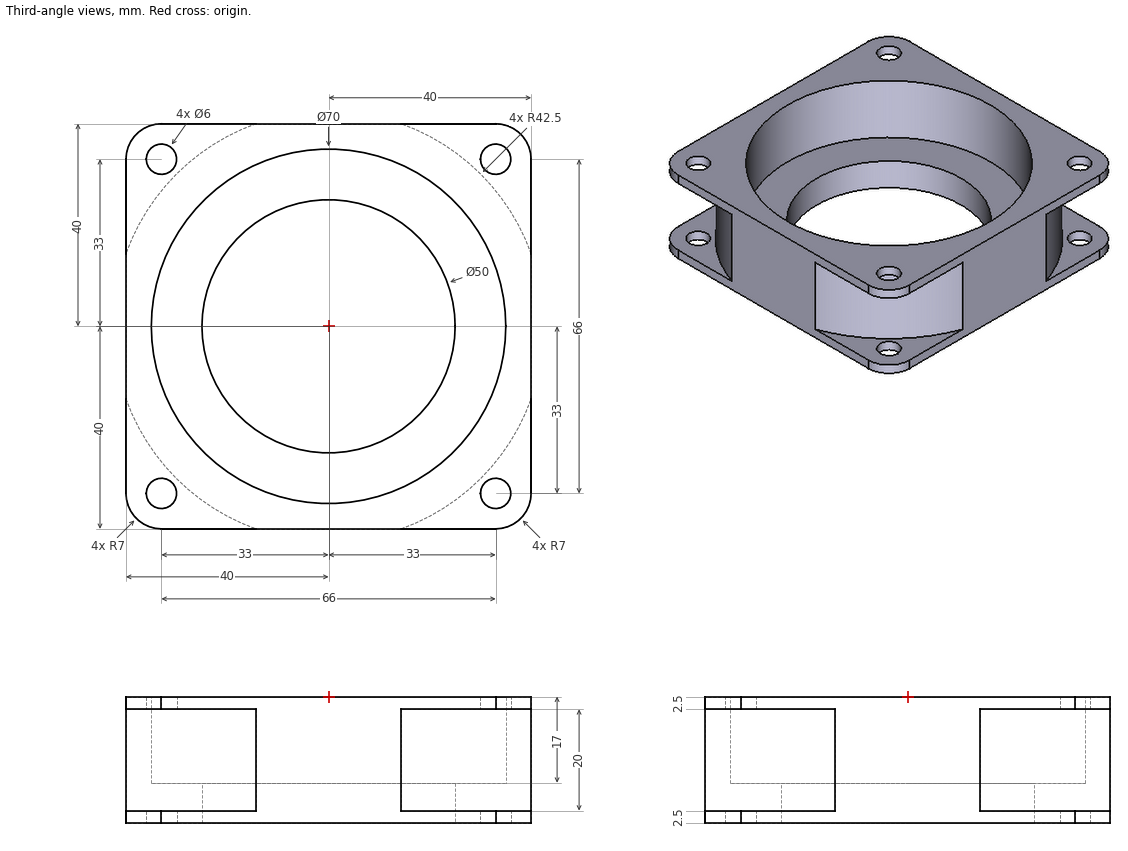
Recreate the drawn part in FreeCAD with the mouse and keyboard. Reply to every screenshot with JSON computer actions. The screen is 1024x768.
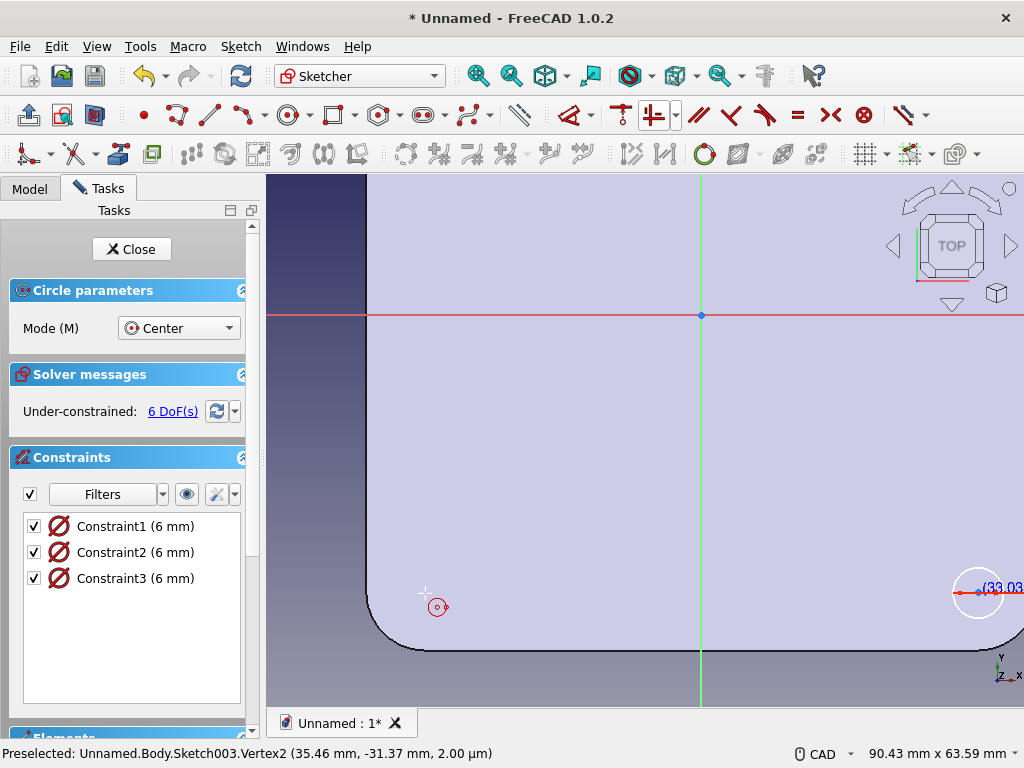
{"action": "left_click", "coordinate": [425, 592]}
{"action": "mouse_move", "coordinate": [443, 574]}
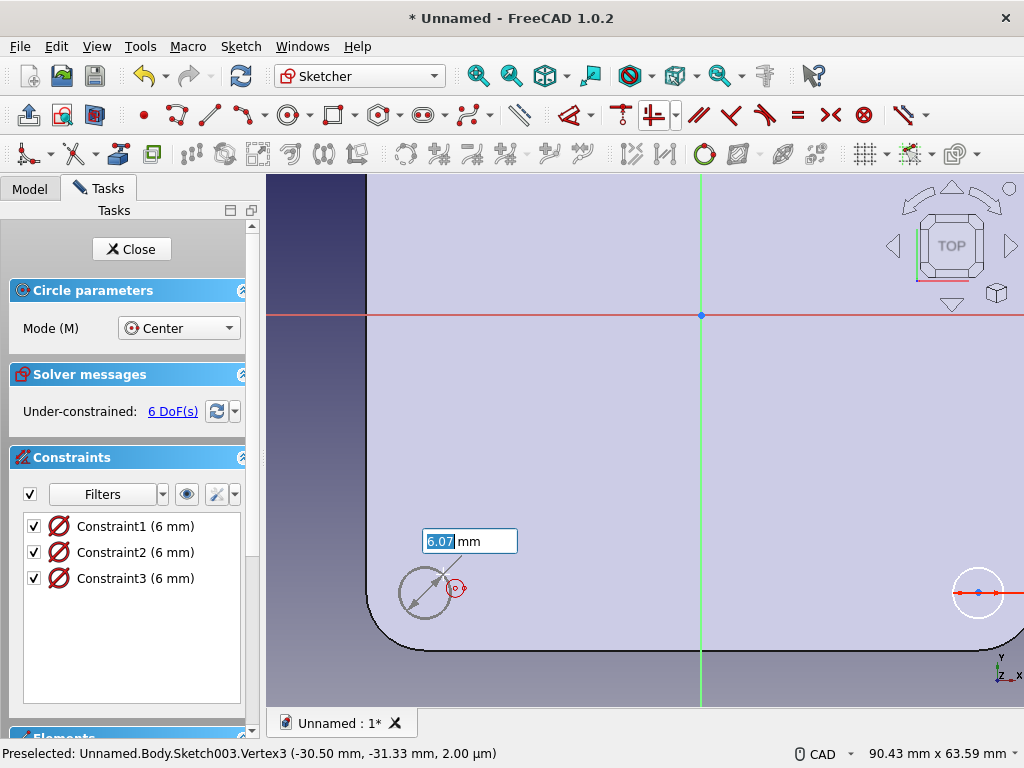
{"action": "type", "text": "6"}
{"action": "key", "text": "Return"}
{"action": "key", "text": "Escape"}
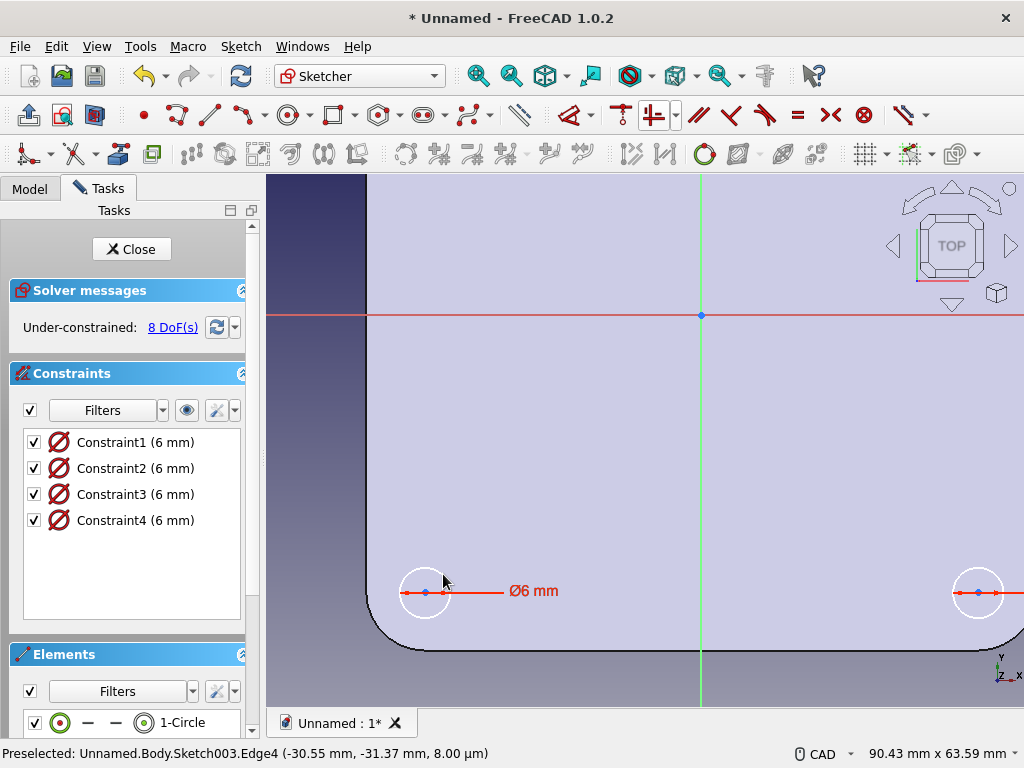
{"action": "scroll", "coordinate": [425, 593], "scroll_direction": "down", "scroll_amount": 3}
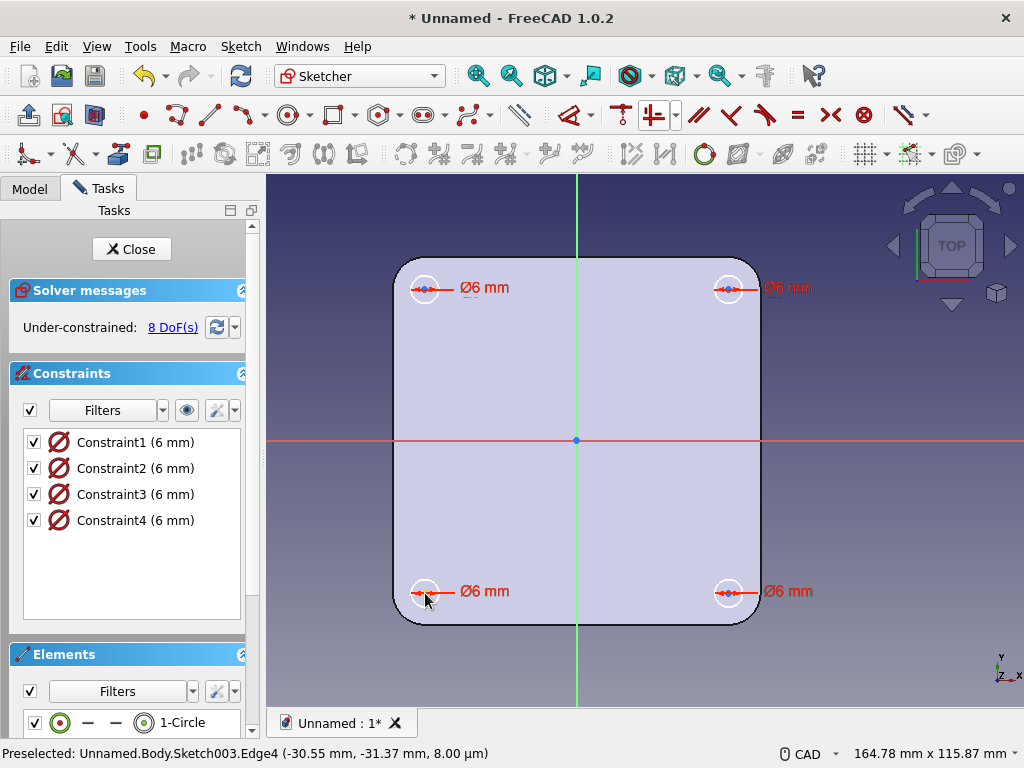
{"action": "left_click", "coordinate": [425, 290]}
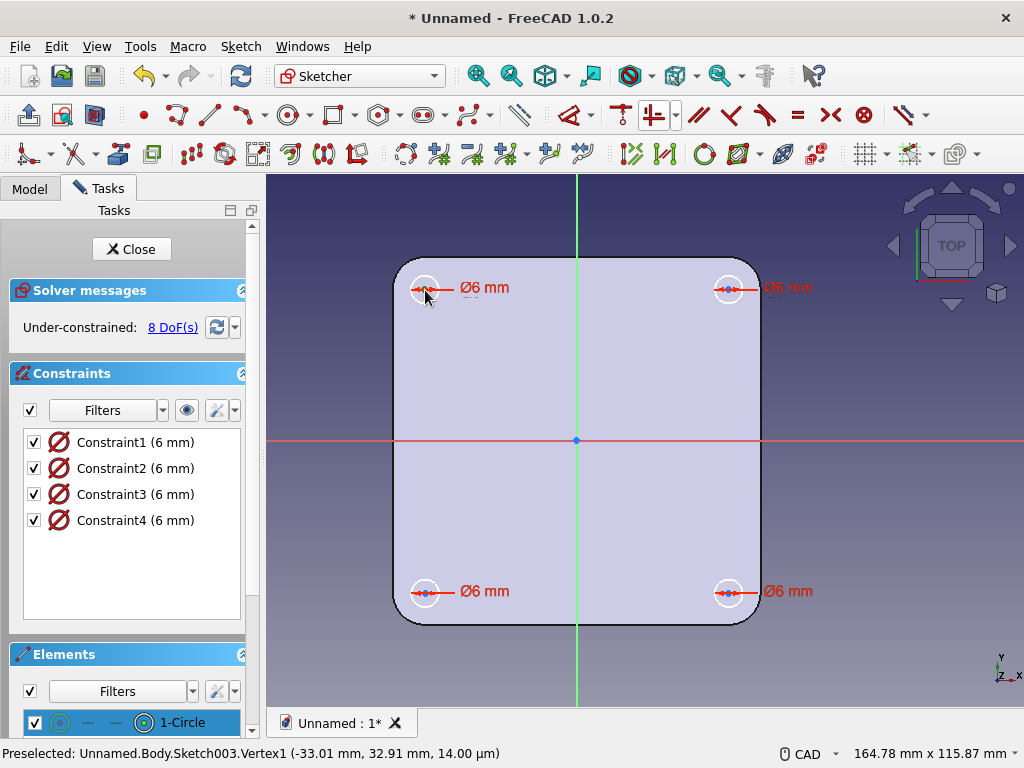
{"action": "left_click", "coordinate": [729, 290]}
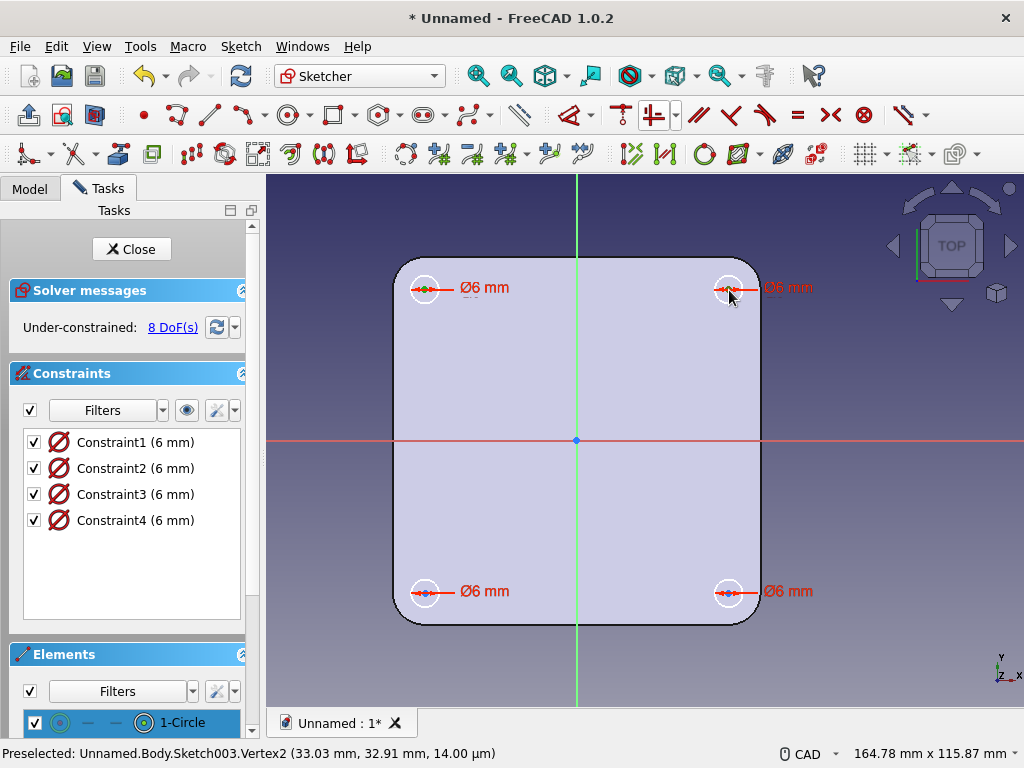
{"action": "key", "text": "h"}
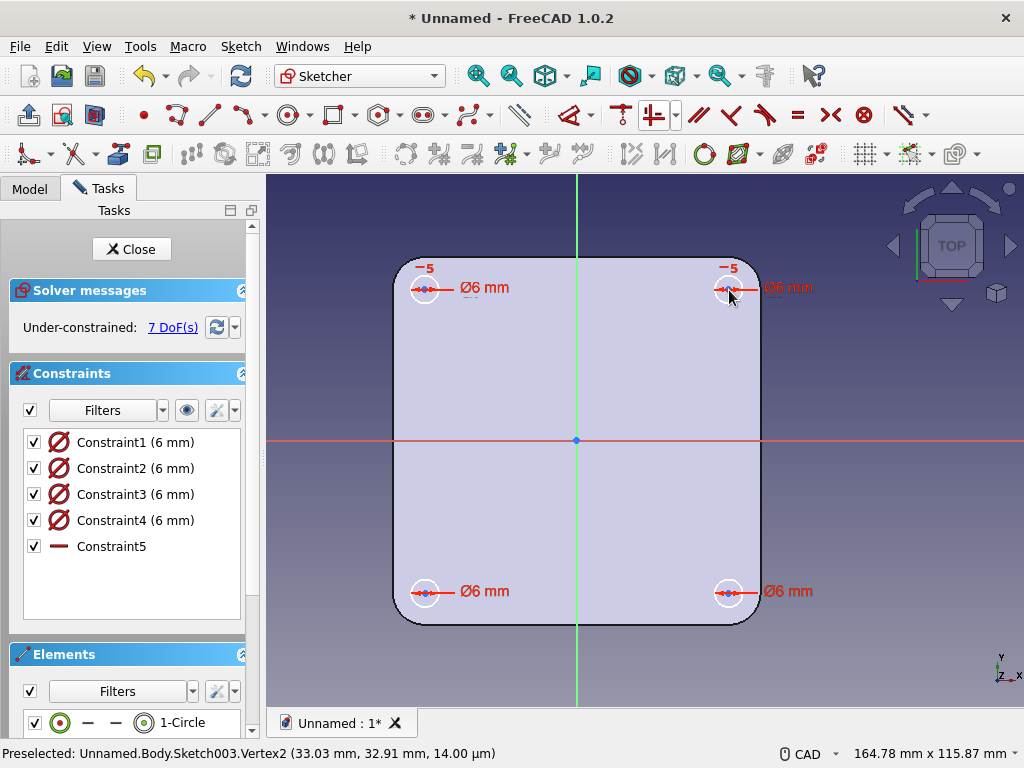
{"action": "left_click", "coordinate": [729, 290]}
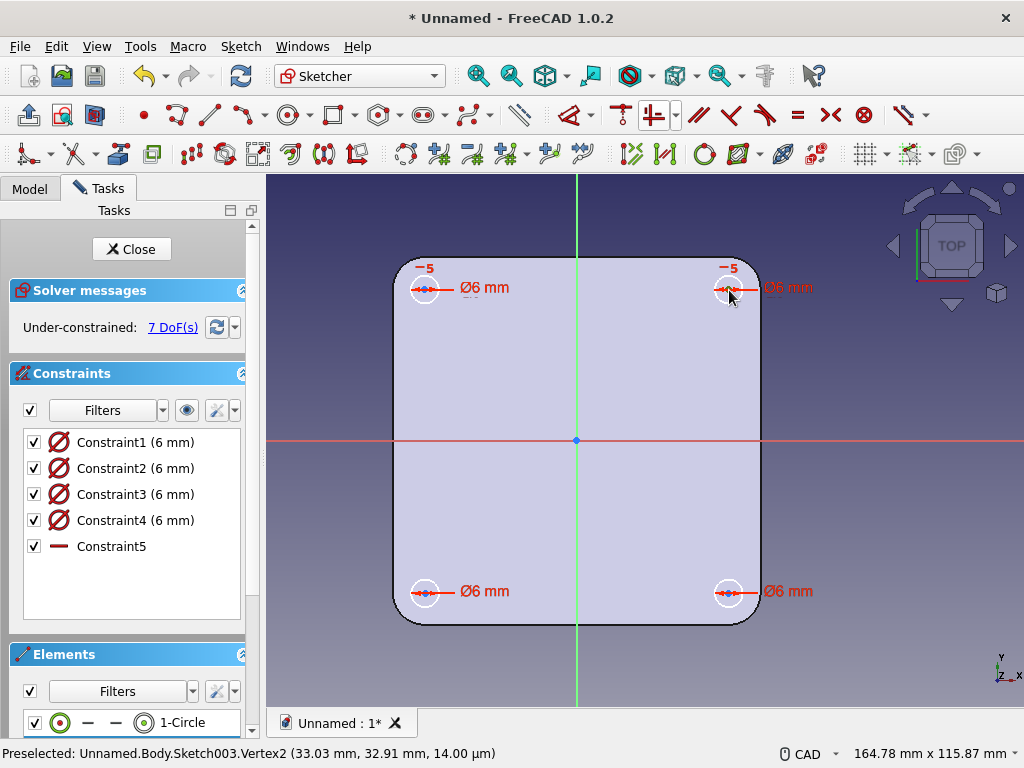
{"action": "left_click", "coordinate": [729, 593]}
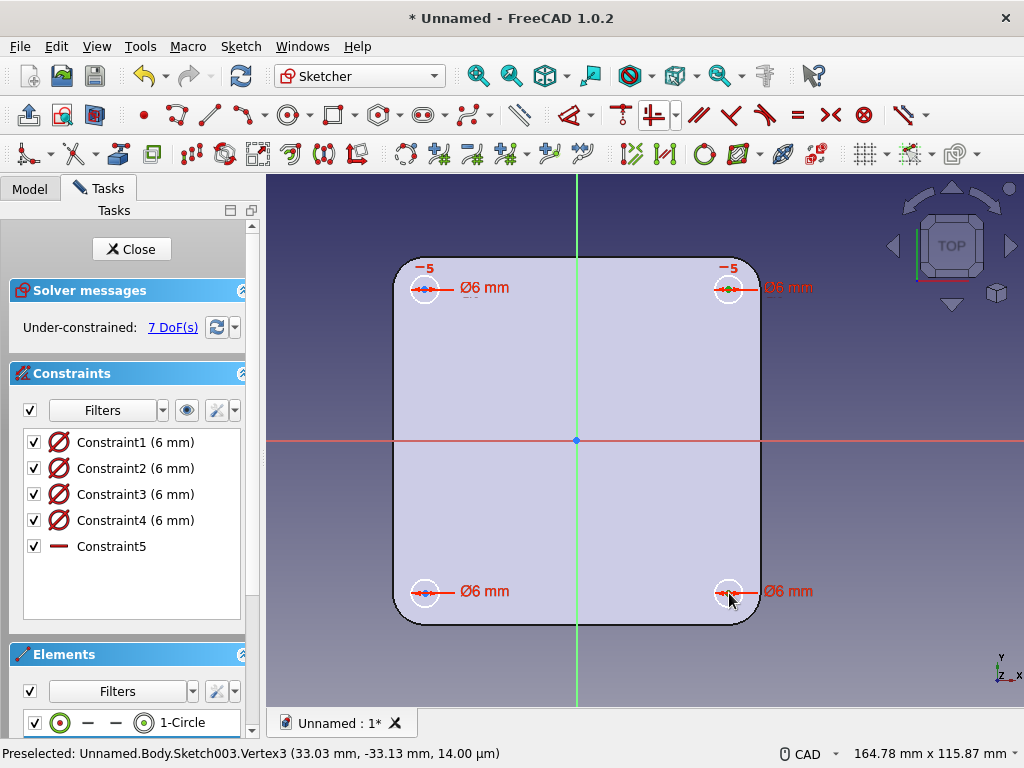
{"action": "key", "text": "v"}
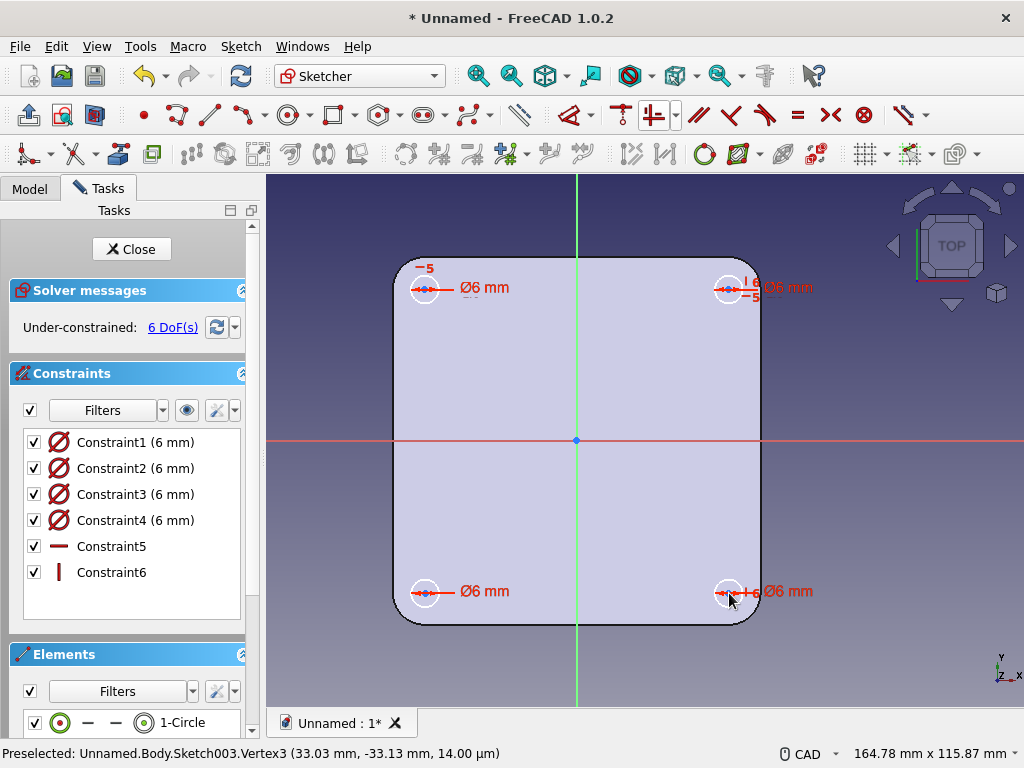
{"action": "left_click", "coordinate": [425, 290]}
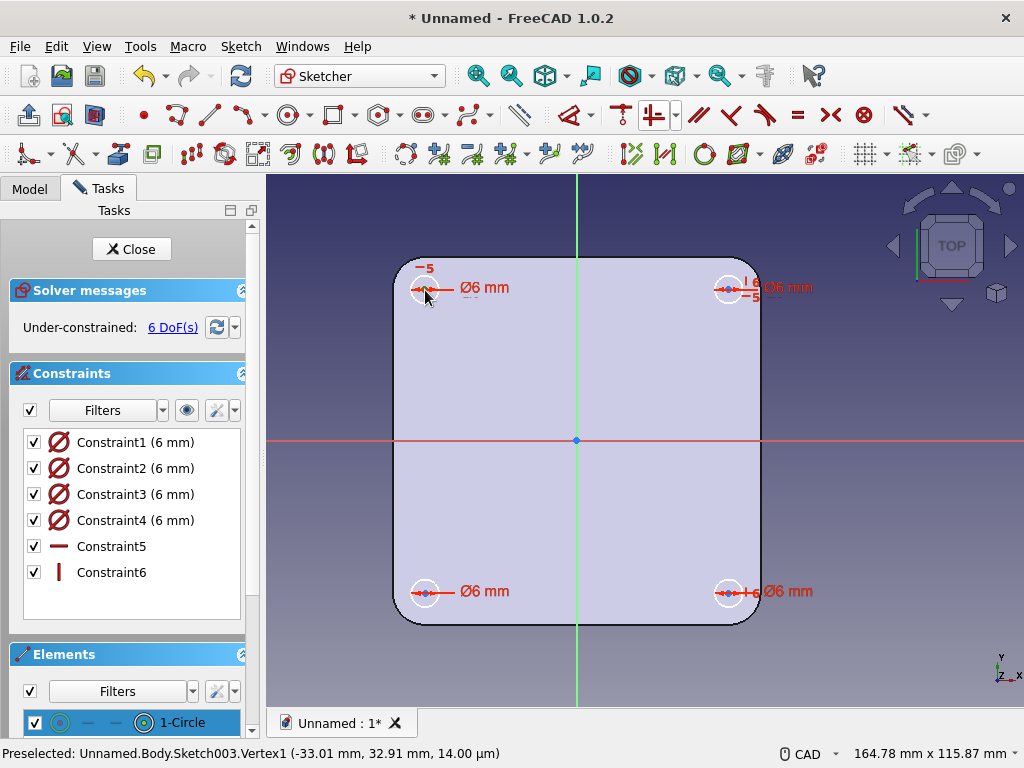
{"action": "left_click", "coordinate": [425, 593]}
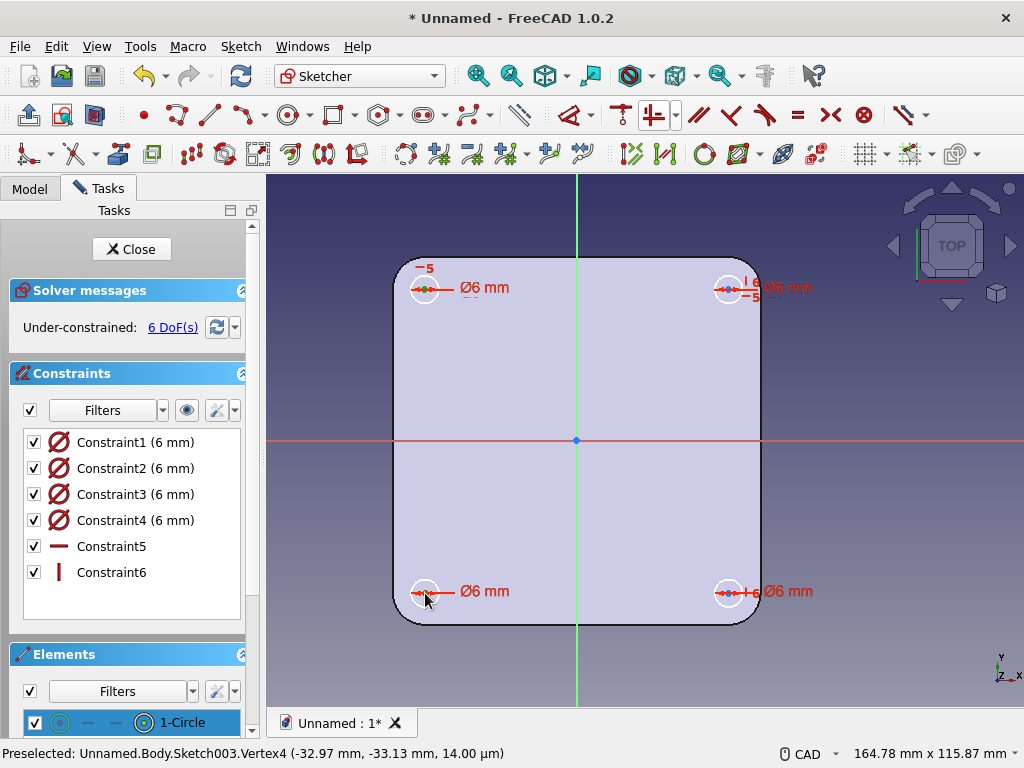
{"action": "left_click", "coordinate": [676, 116]}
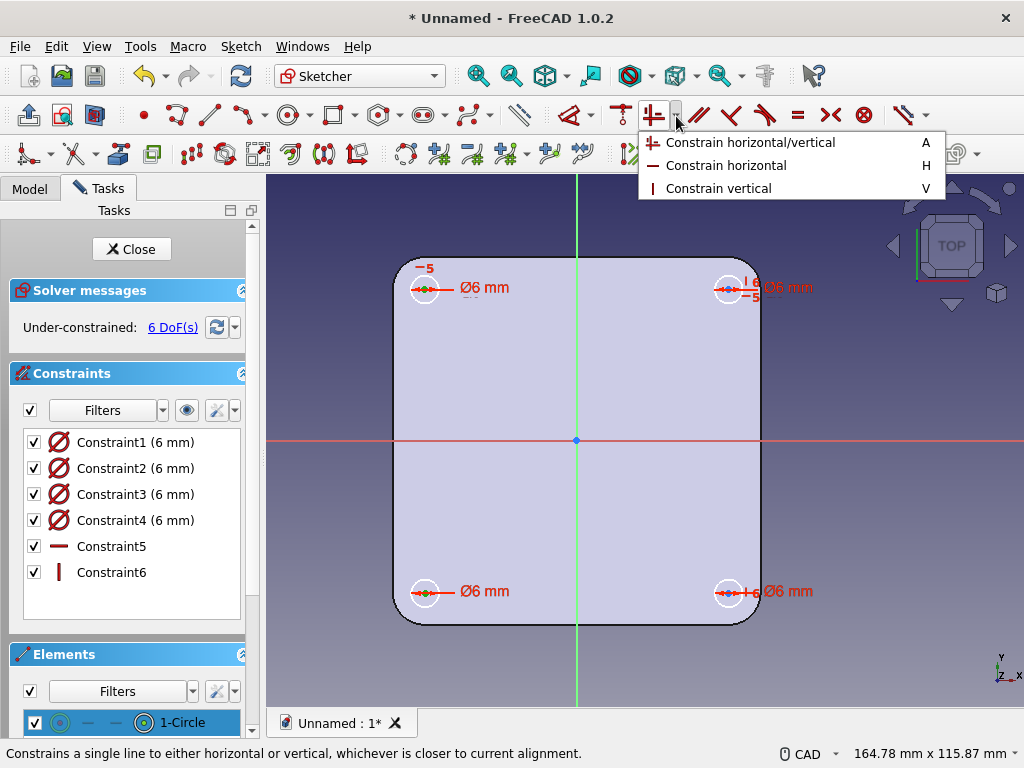
{"action": "left_click", "coordinate": [792, 188]}